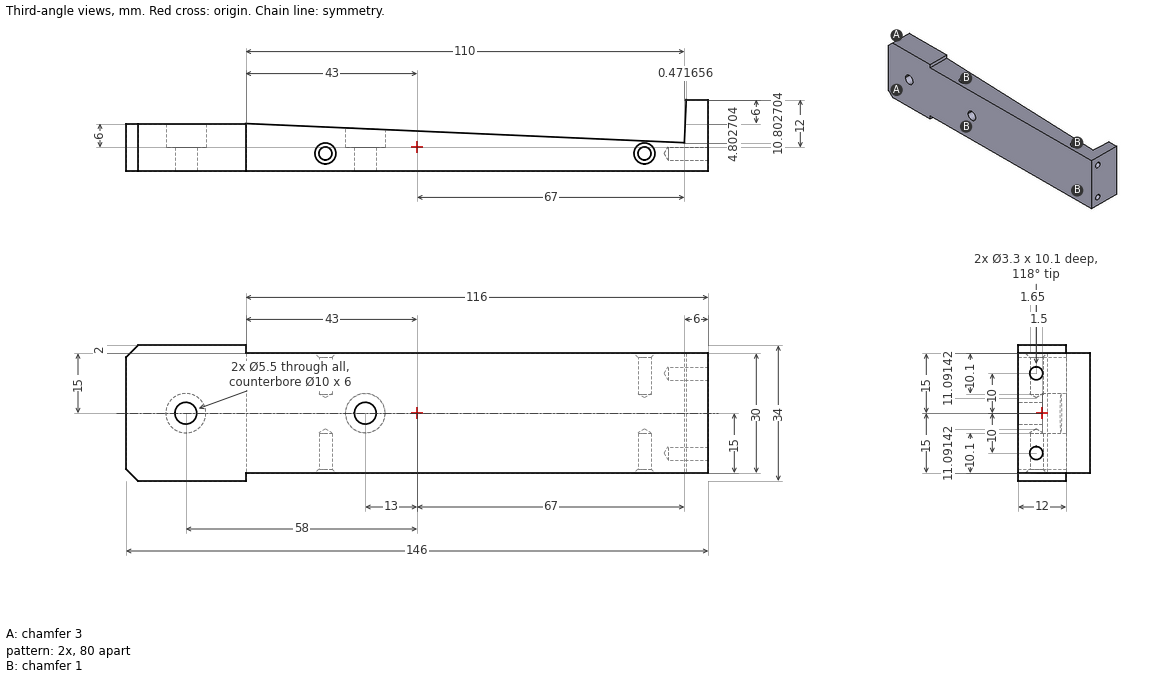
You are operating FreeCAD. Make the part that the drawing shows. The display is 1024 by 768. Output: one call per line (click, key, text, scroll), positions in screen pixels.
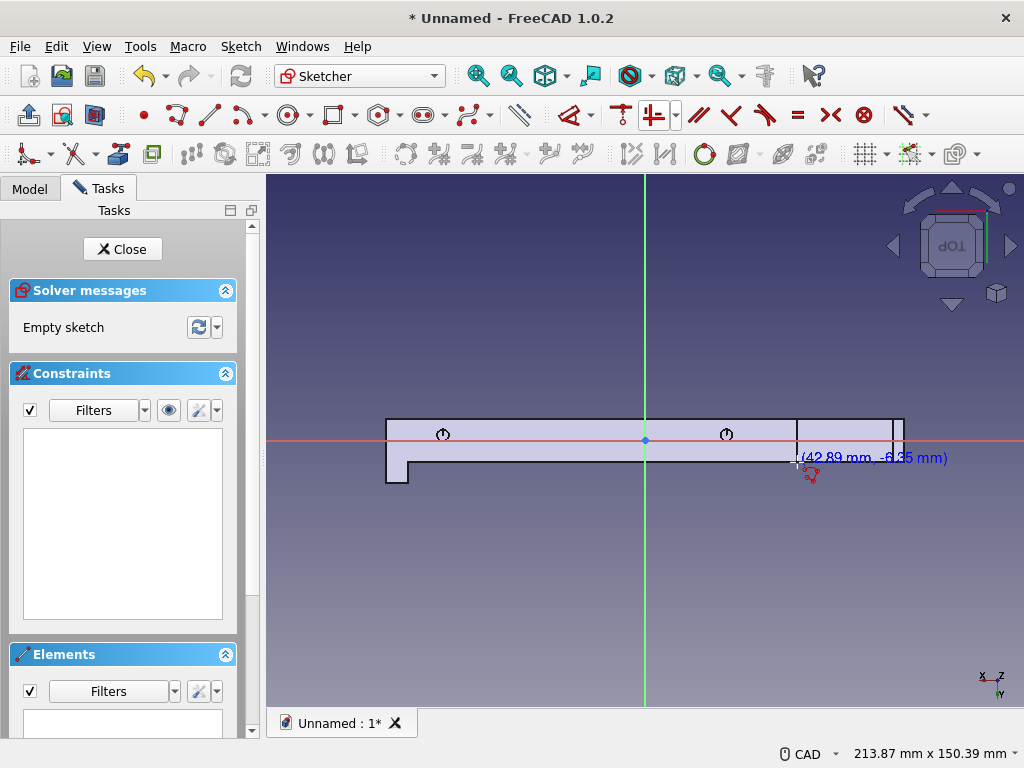
scroll(408, 445, up, 7)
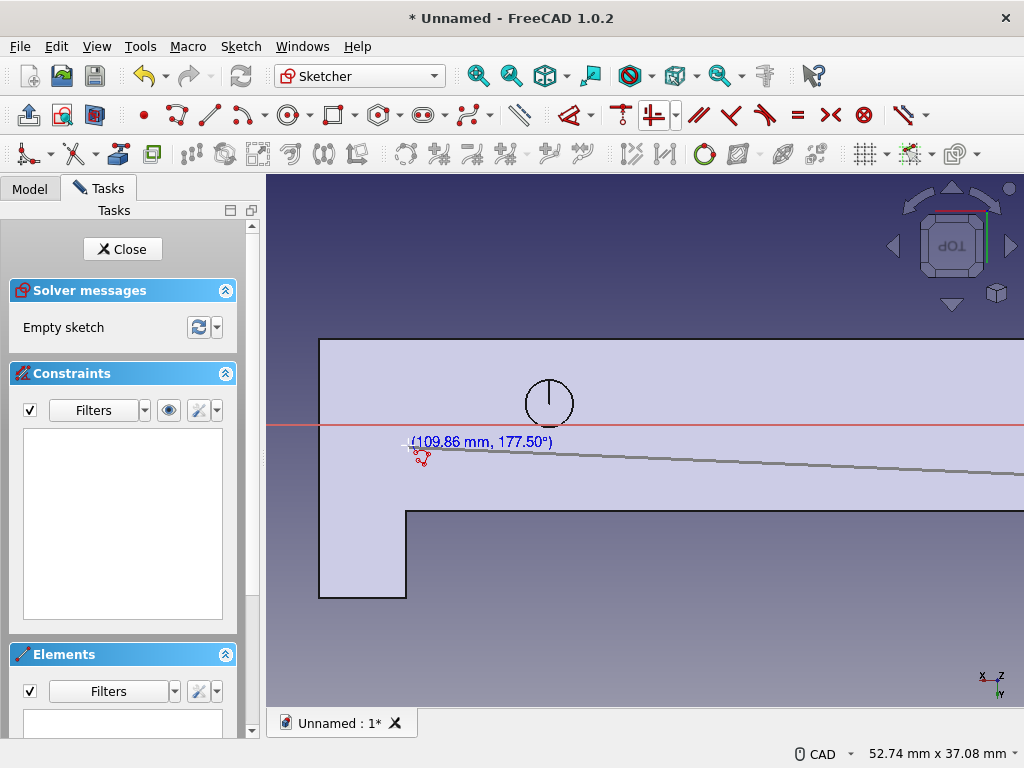
click(406, 440)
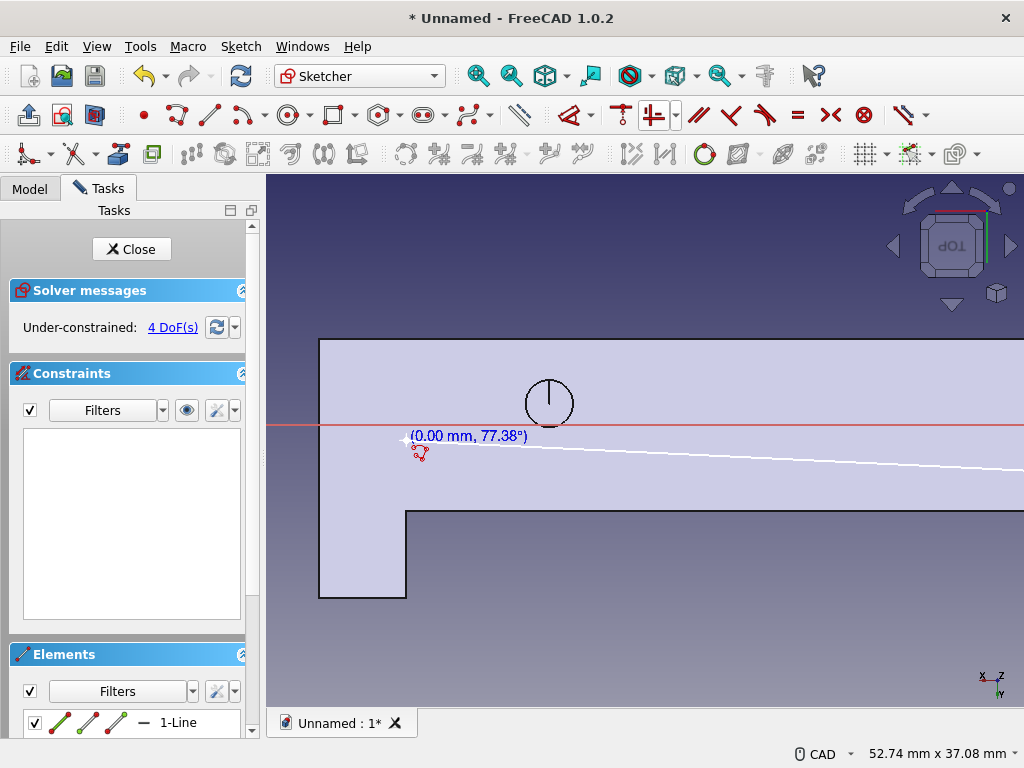
scroll(374, 431, down, 7)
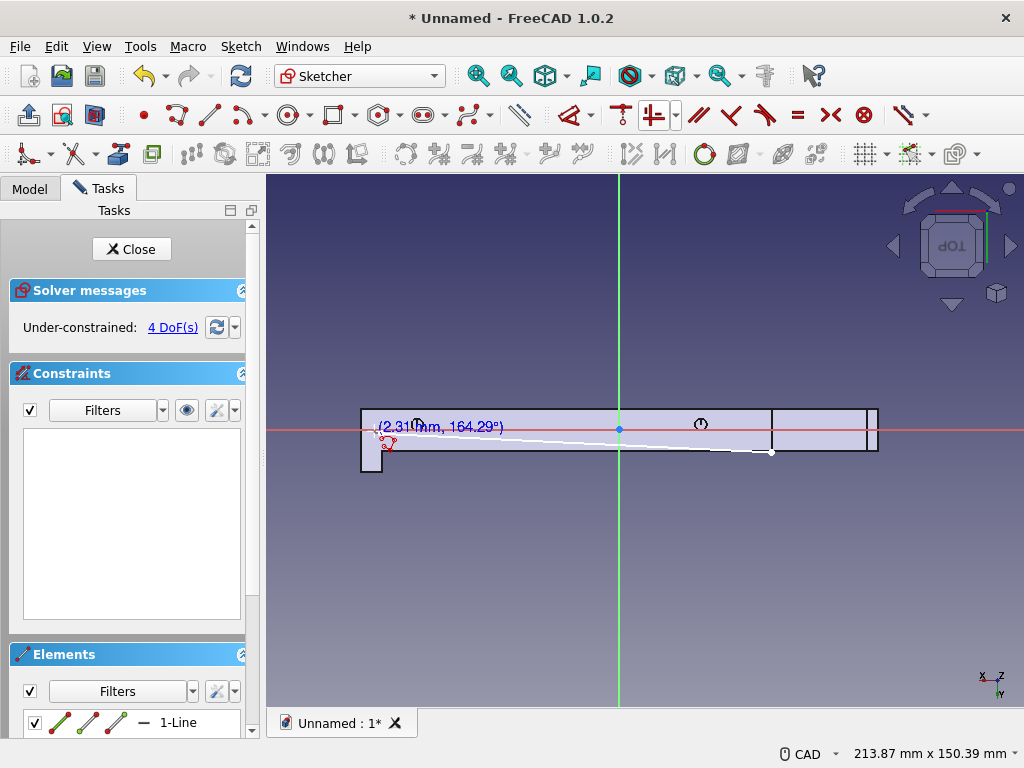
click(382, 451)
click(771, 452)
key(Escape)
key(Escape)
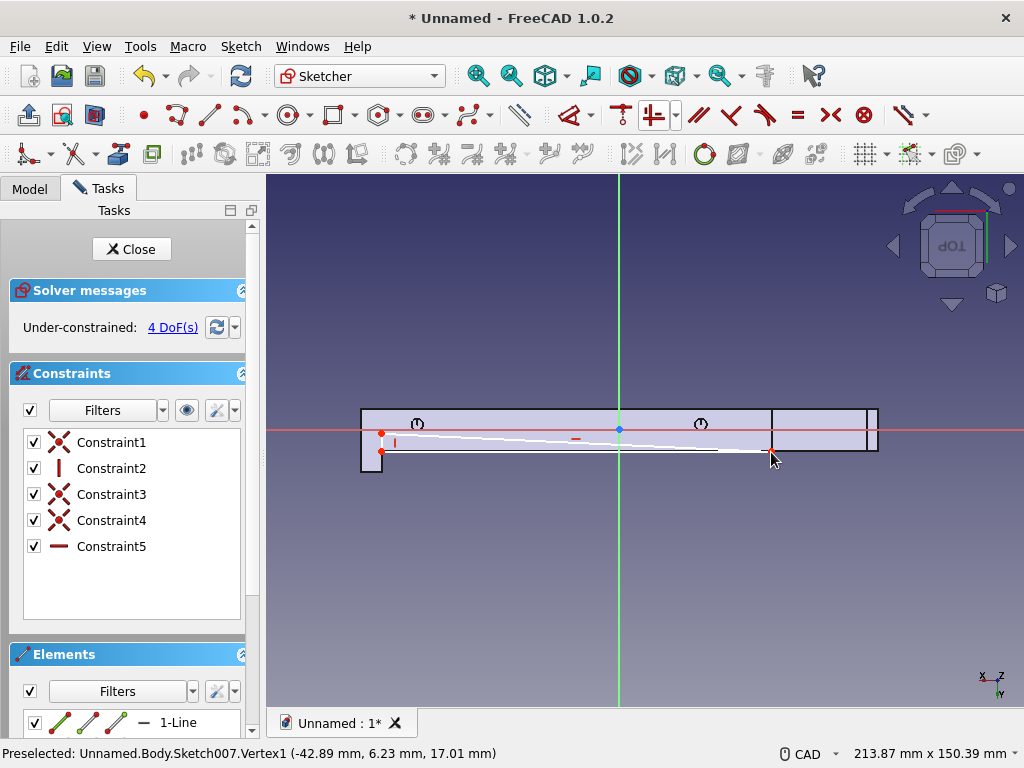
key(d)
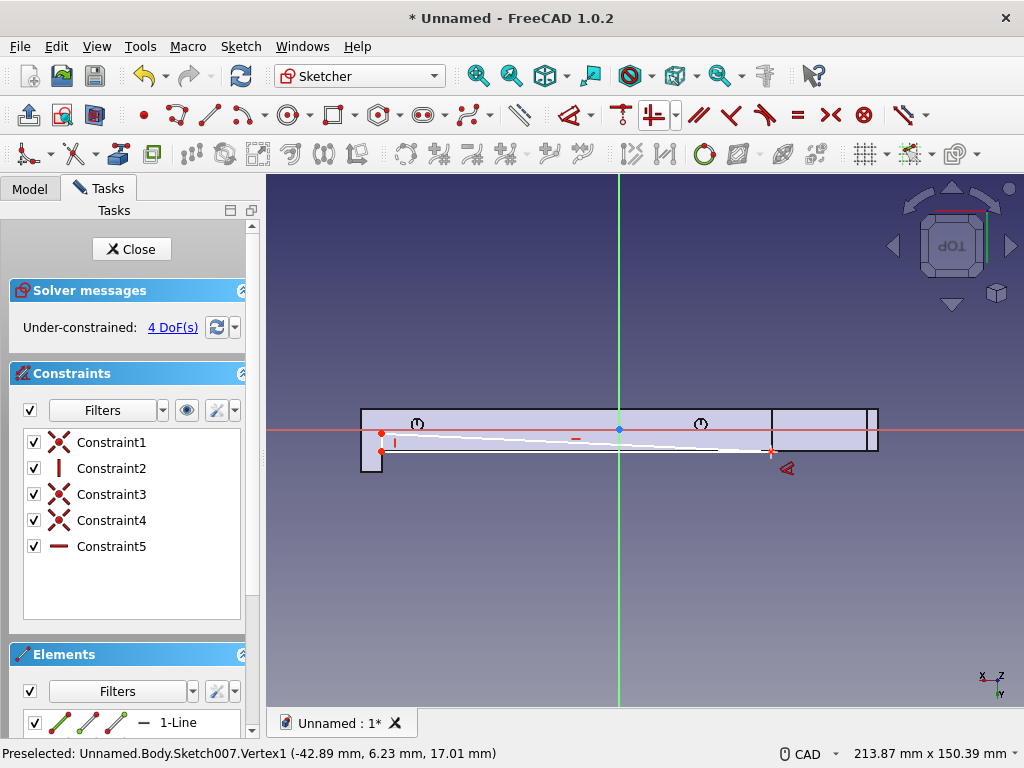
scroll(771, 452, up, 4)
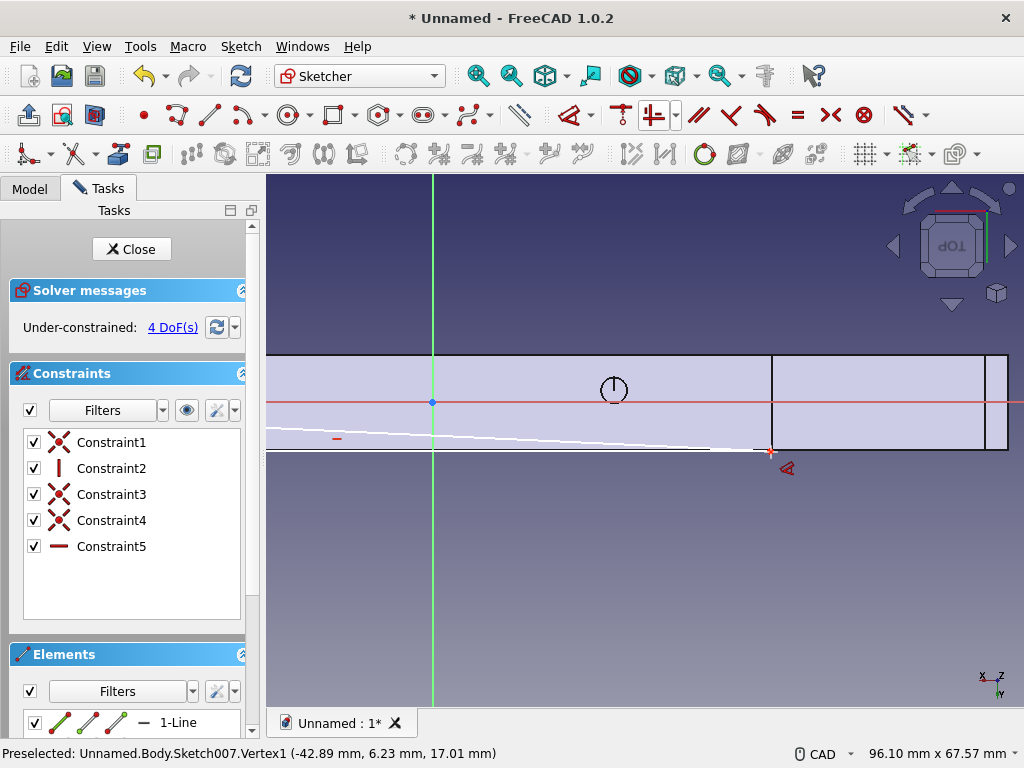
click(771, 451)
click(805, 427)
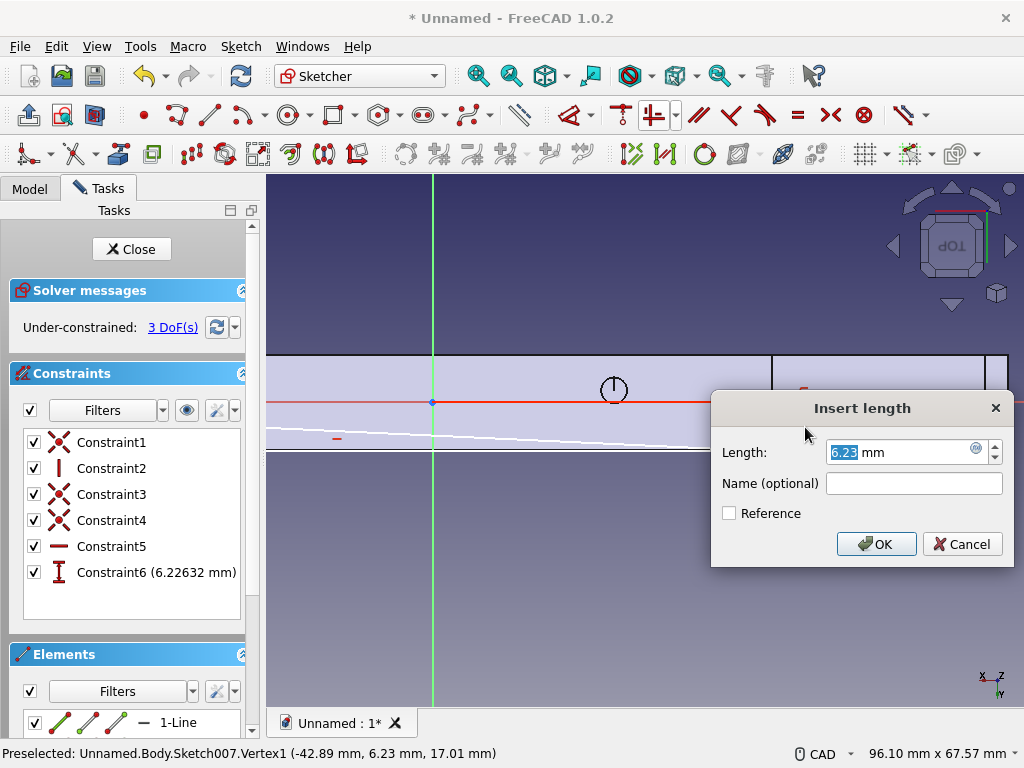
text(6)
key(Return)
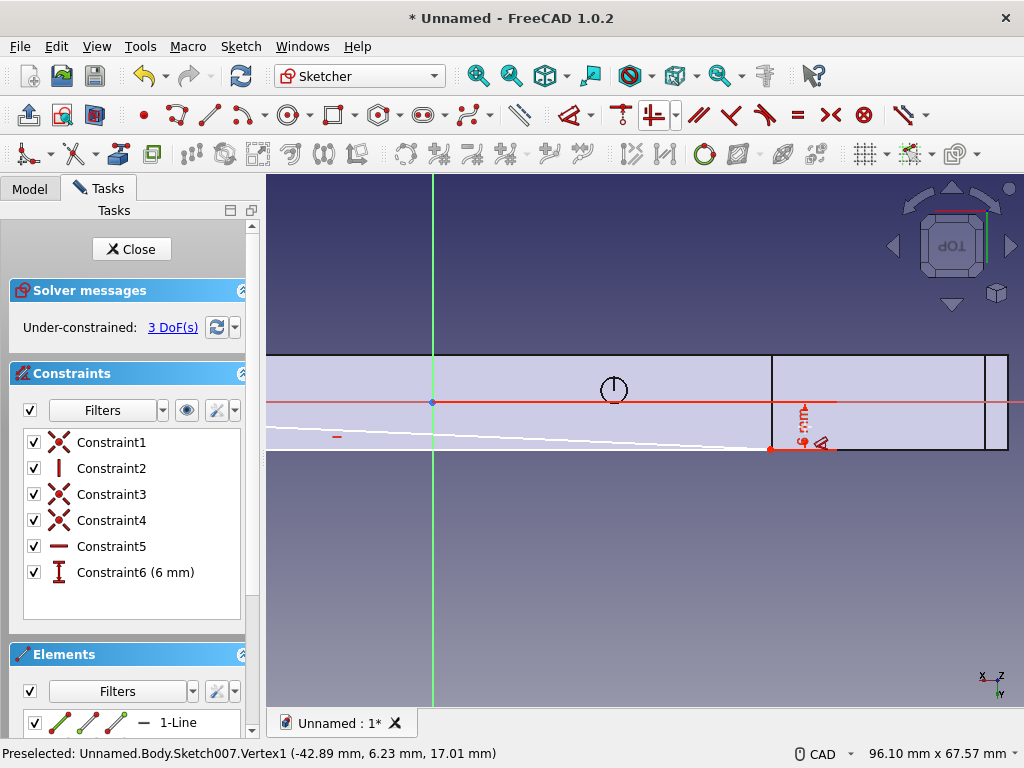
click(511, 450)
click(532, 484)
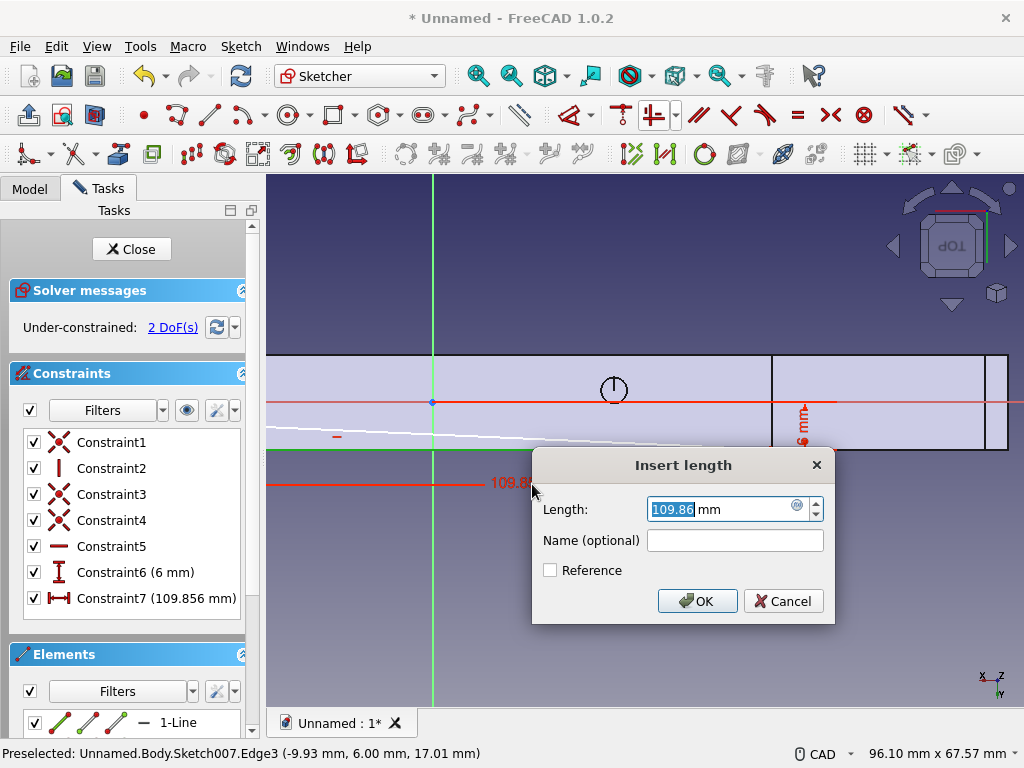
text(110)
key(Return)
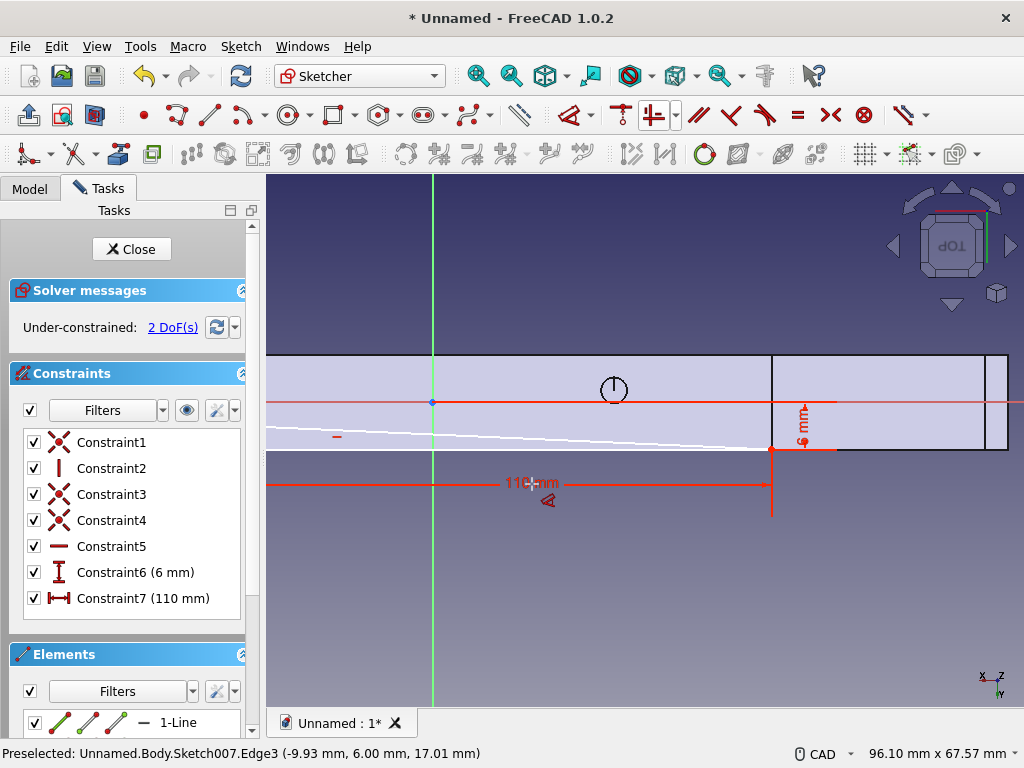
click(772, 450)
click(680, 484)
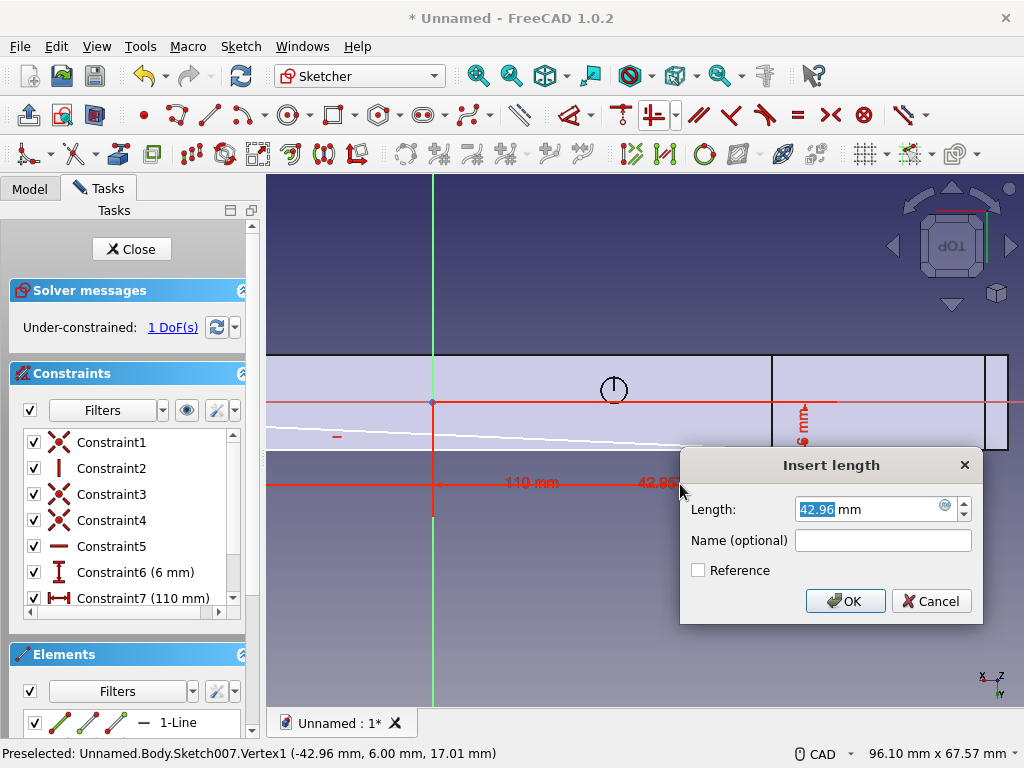
text(43)
key(Return)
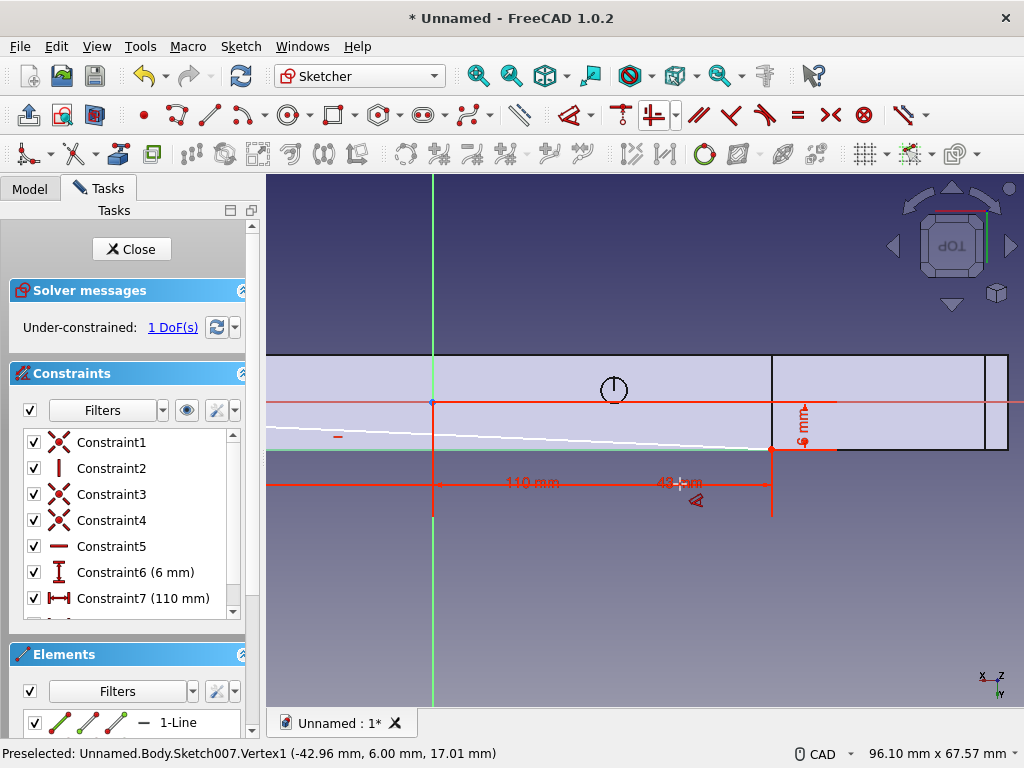
scroll(771, 452, down, 4)